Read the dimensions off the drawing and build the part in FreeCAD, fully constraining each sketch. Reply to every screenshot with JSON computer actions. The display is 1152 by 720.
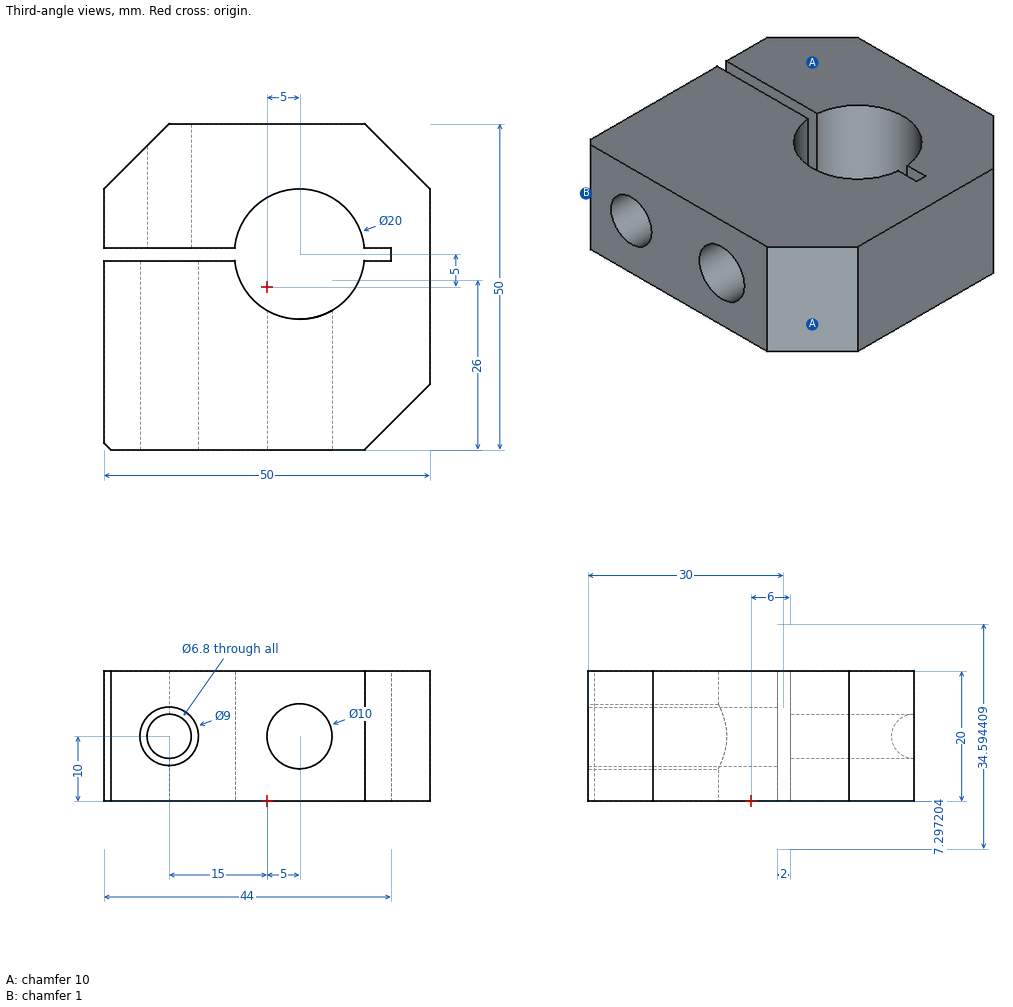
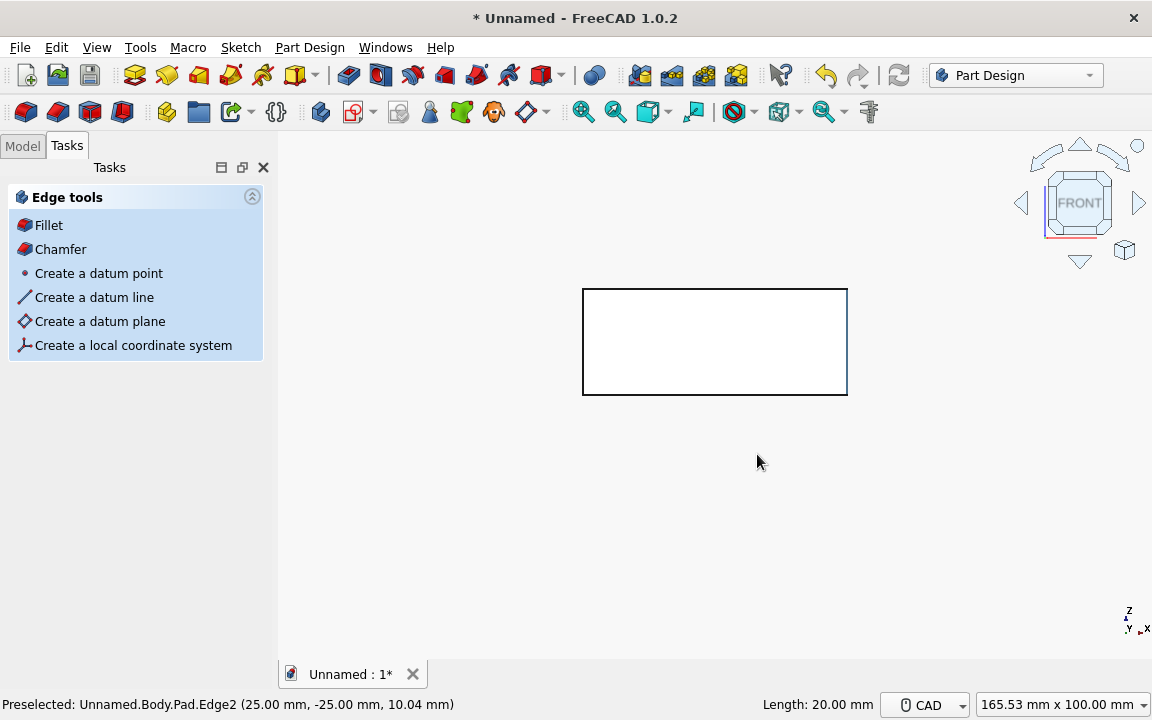
{"action": "left_click", "coordinate": [584, 112]}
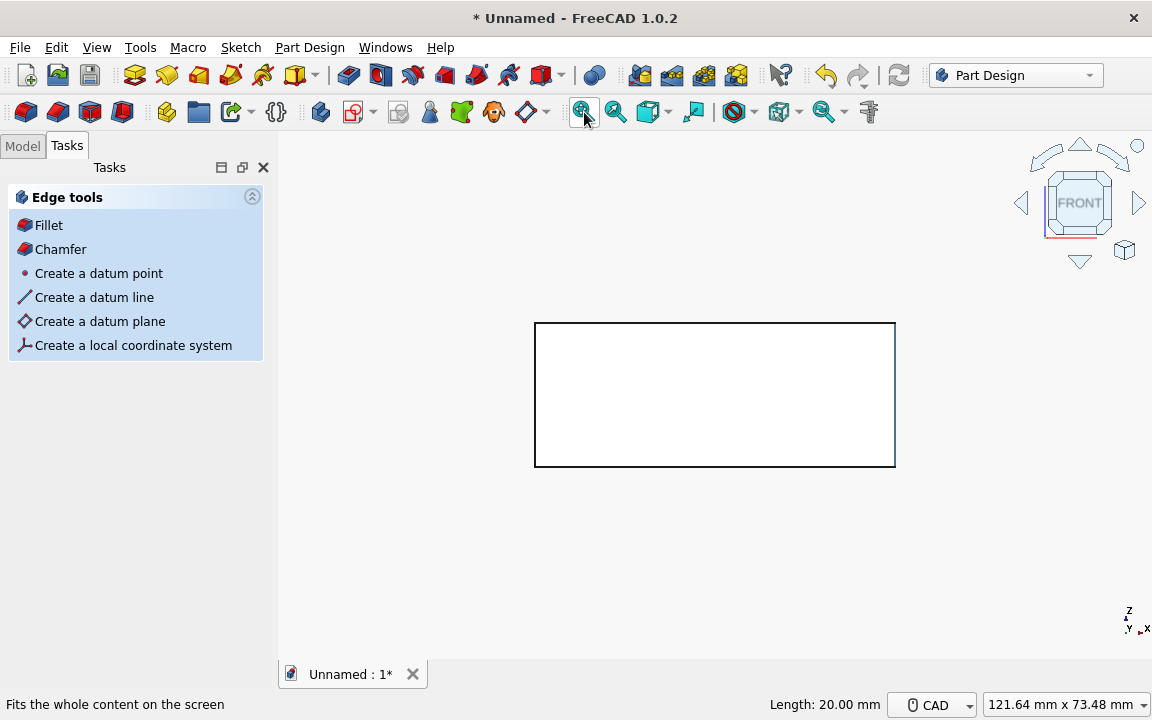
{"action": "key", "text": "3"}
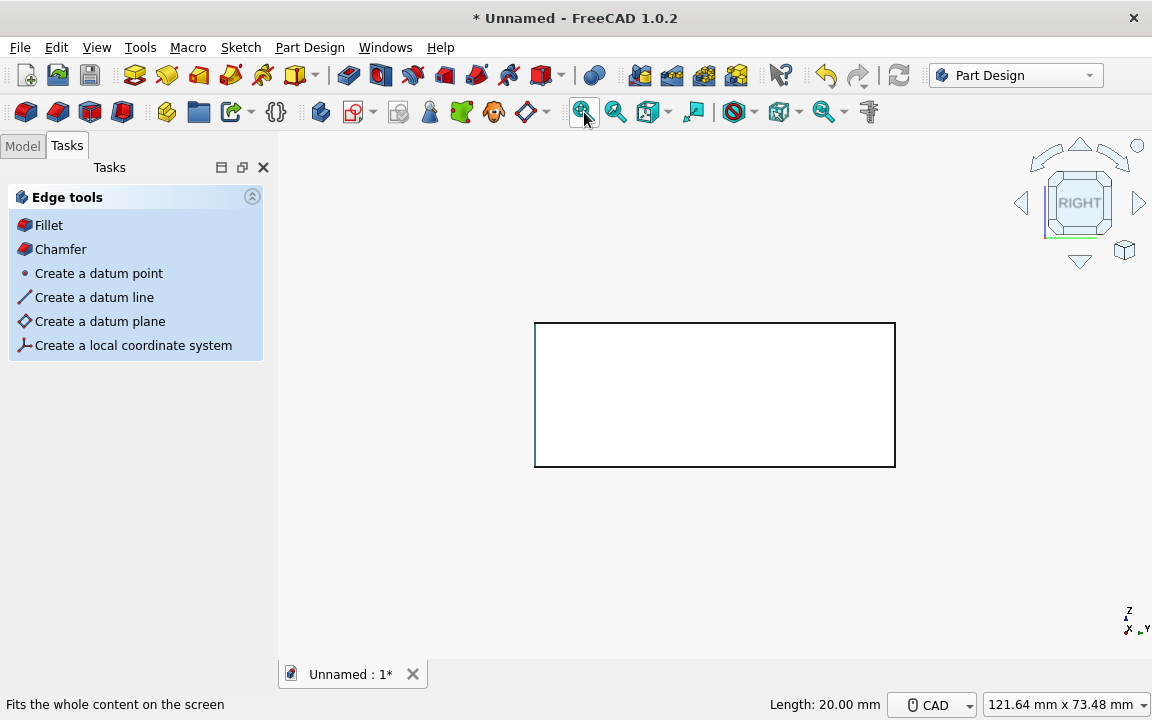
{"action": "left_click", "coordinate": [584, 112]}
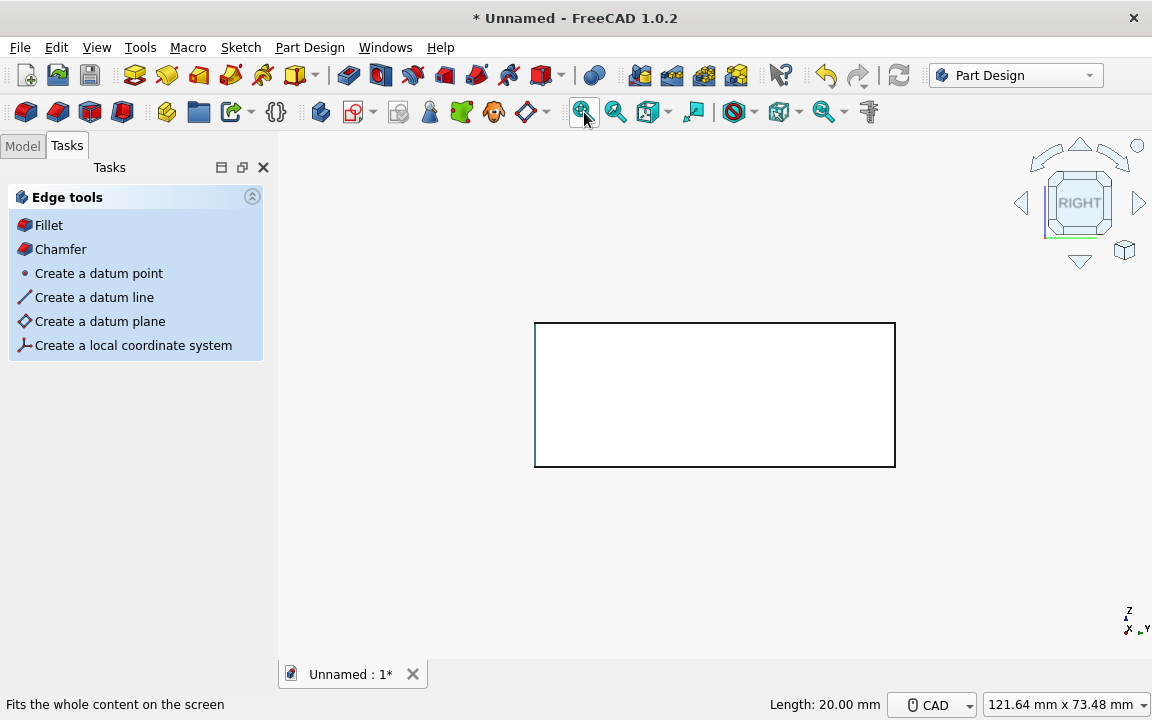
{"action": "left_click", "coordinate": [895, 394], "text": "ctrl"}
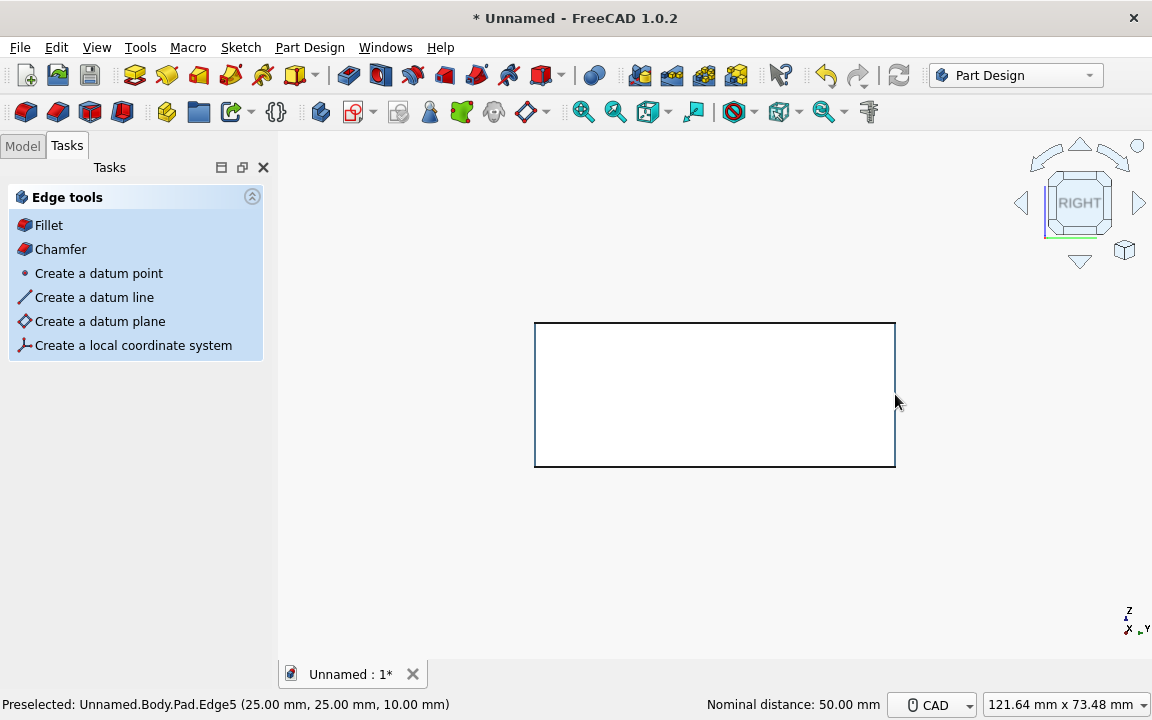
{"action": "key", "text": "5"}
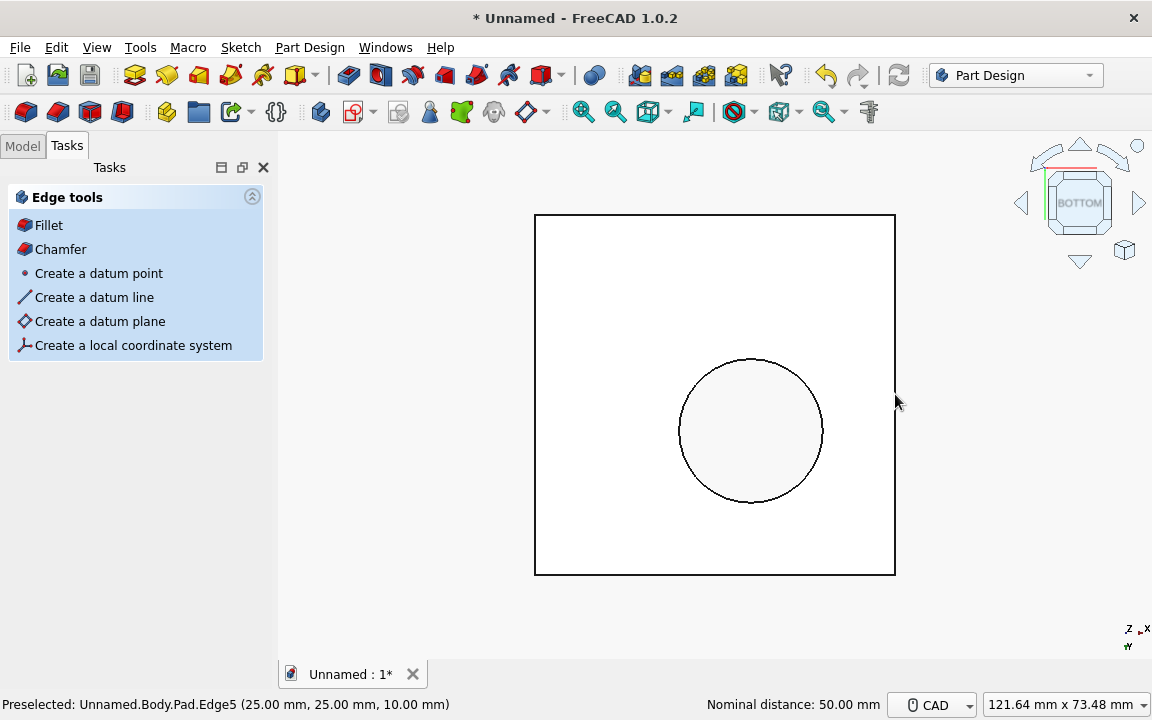
{"action": "key", "text": "4"}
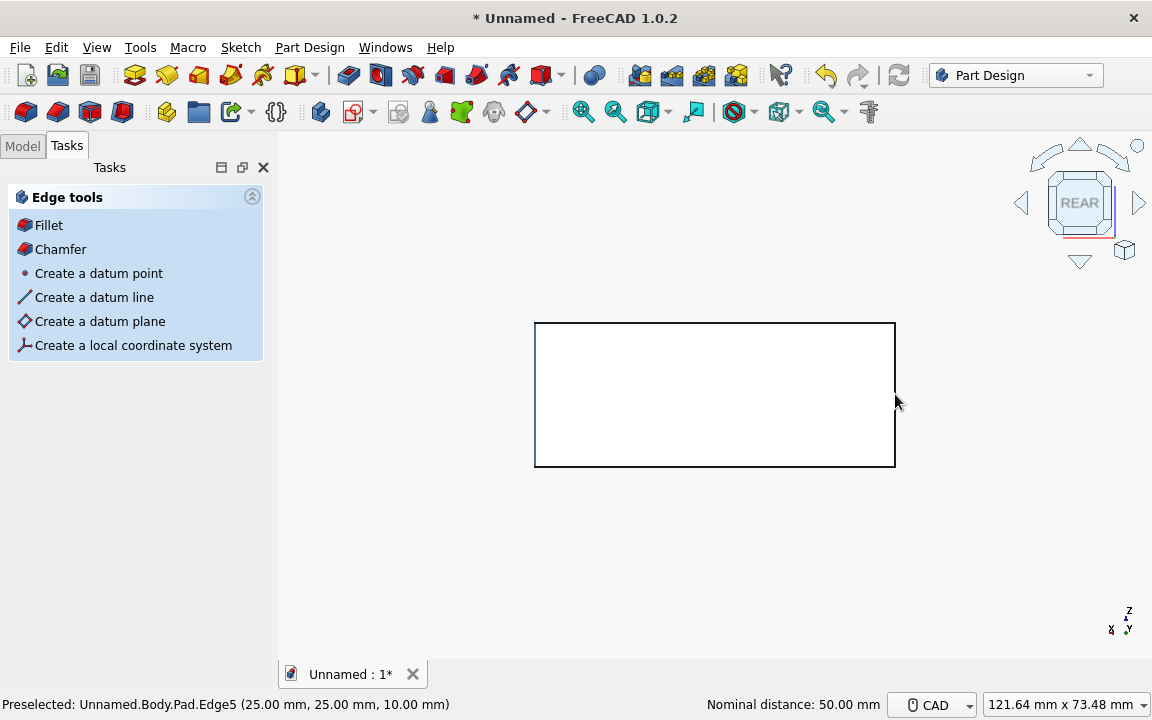
{"action": "left_click", "coordinate": [584, 112]}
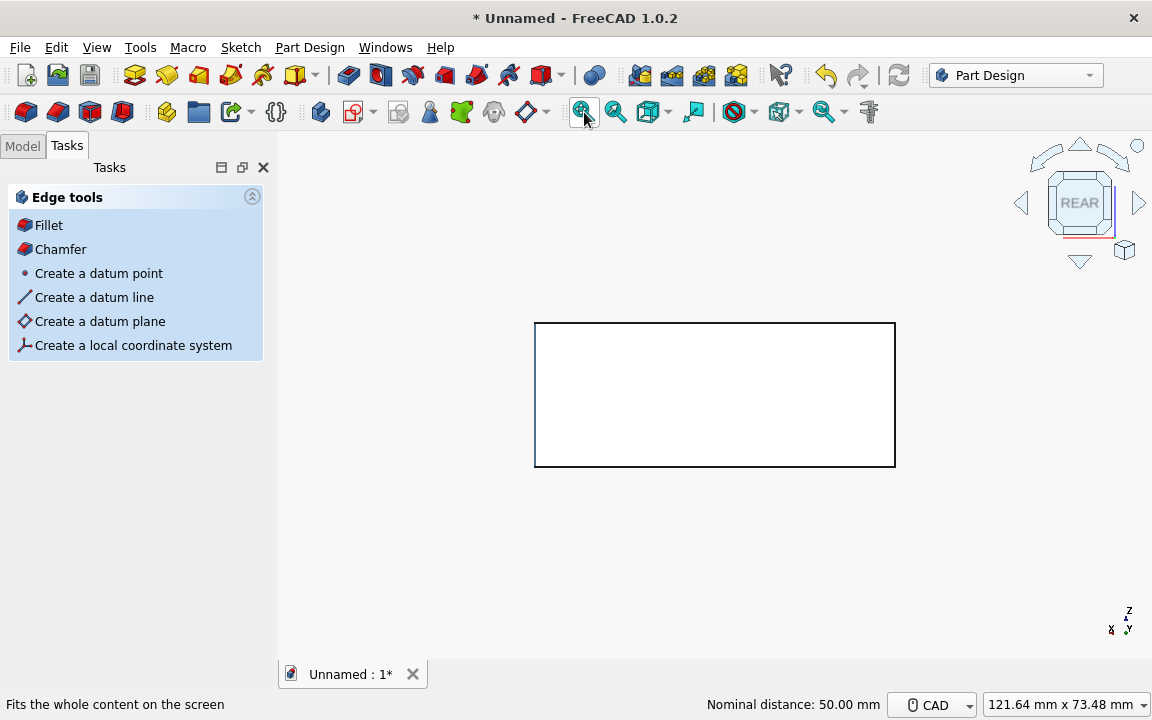
{"action": "left_click", "coordinate": [895, 394], "text": "ctrl"}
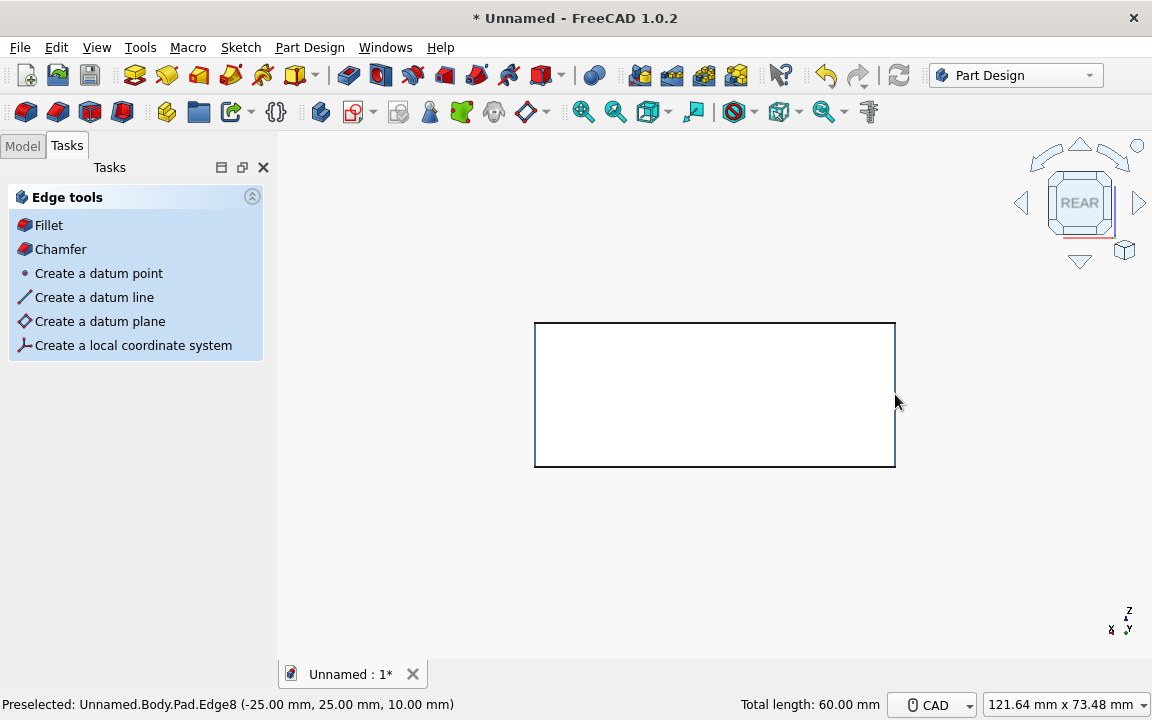
{"action": "left_click", "coordinate": [58, 112]}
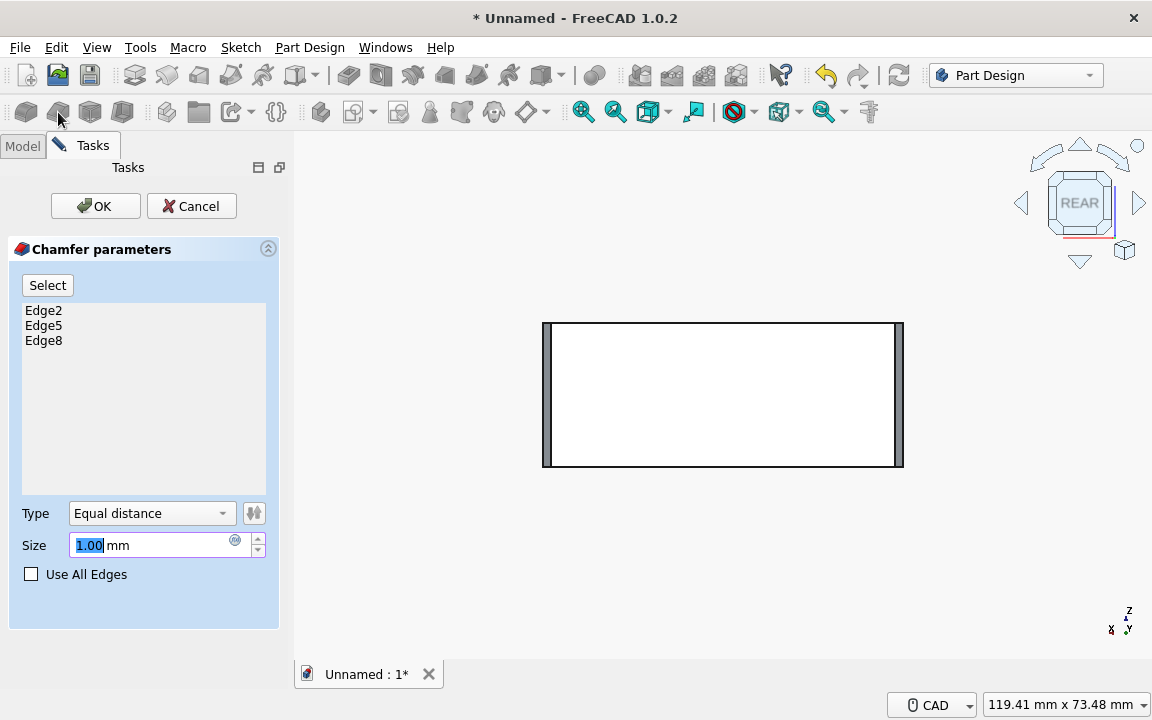
{"action": "type", "text": "10"}
{"action": "key", "text": "Tab"}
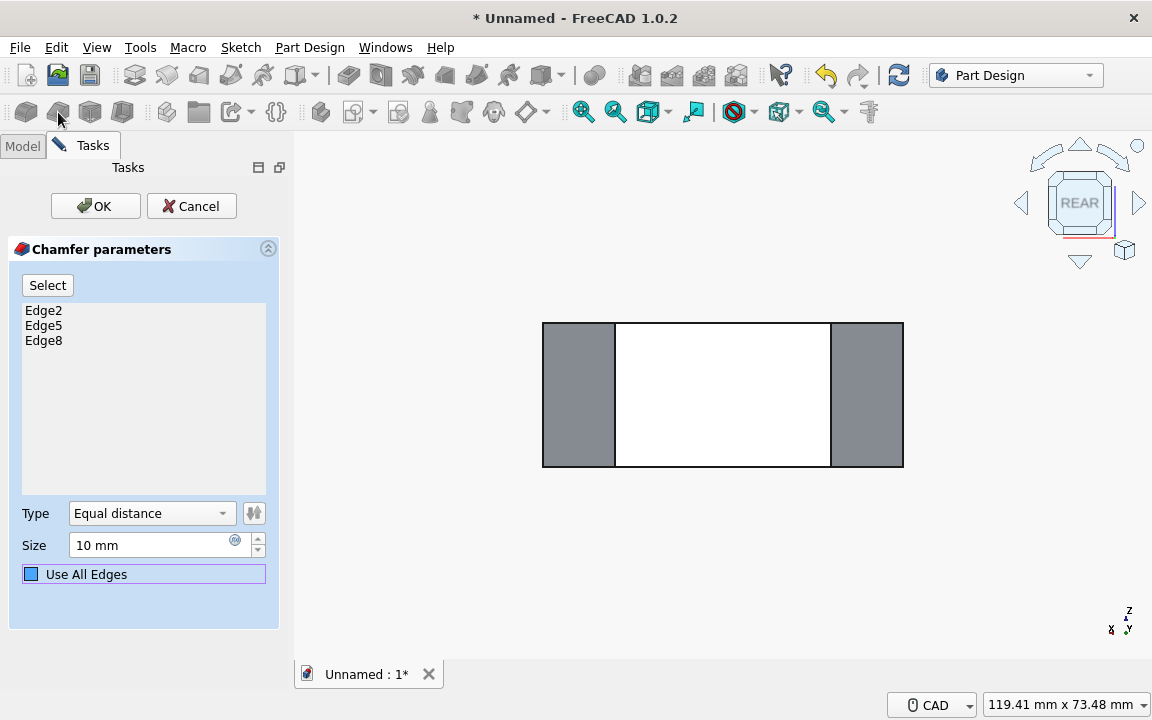
{"action": "left_click", "coordinate": [96, 206]}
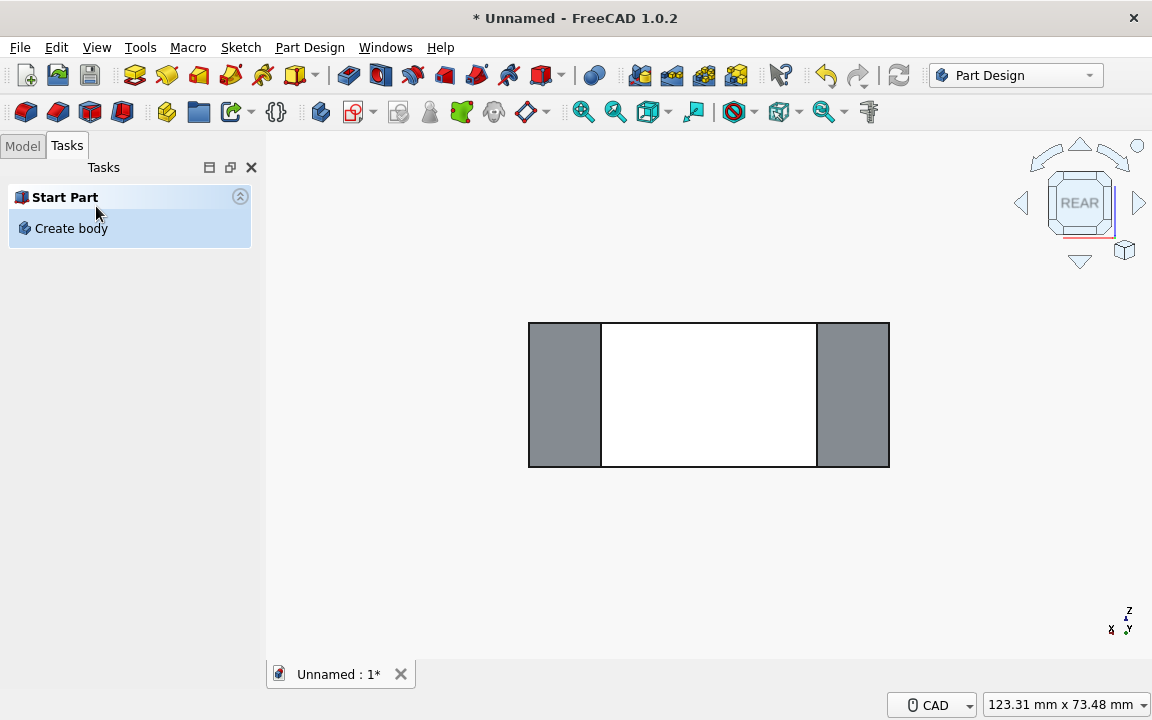
{"action": "left_click", "coordinate": [584, 112]}